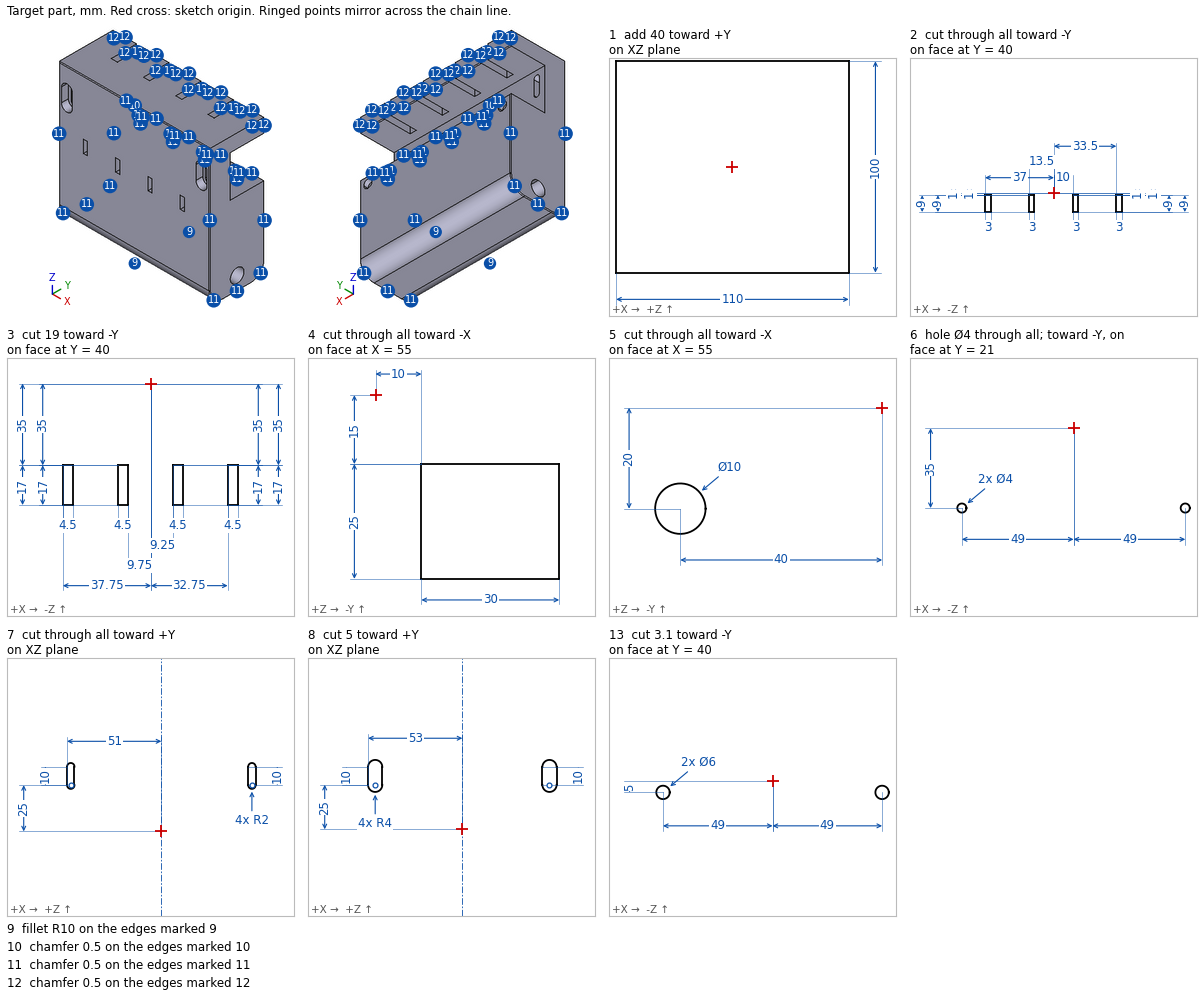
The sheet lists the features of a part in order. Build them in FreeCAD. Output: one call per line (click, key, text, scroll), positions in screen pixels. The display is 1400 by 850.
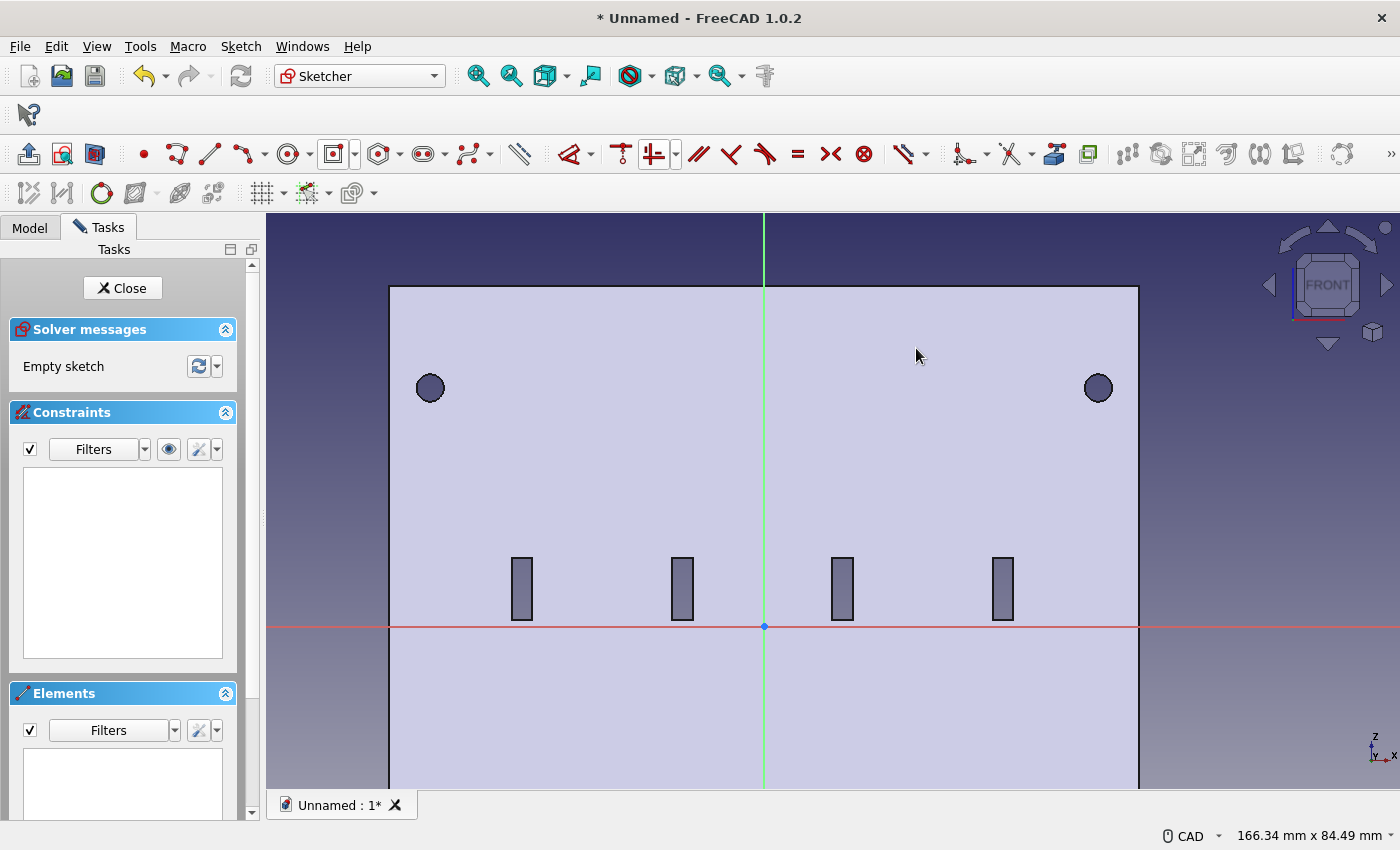
scroll(430, 456, up, 3)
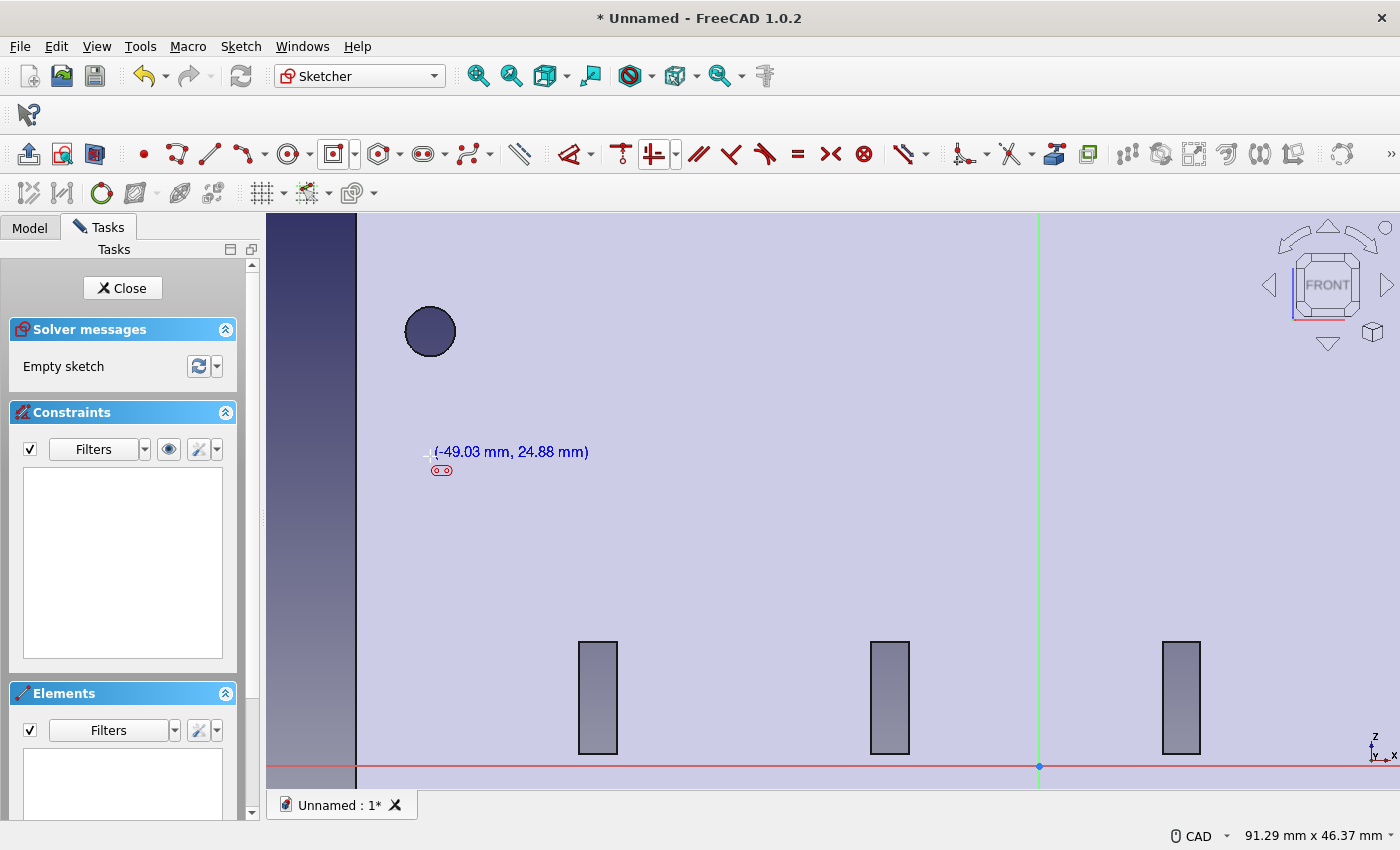
click(430, 456)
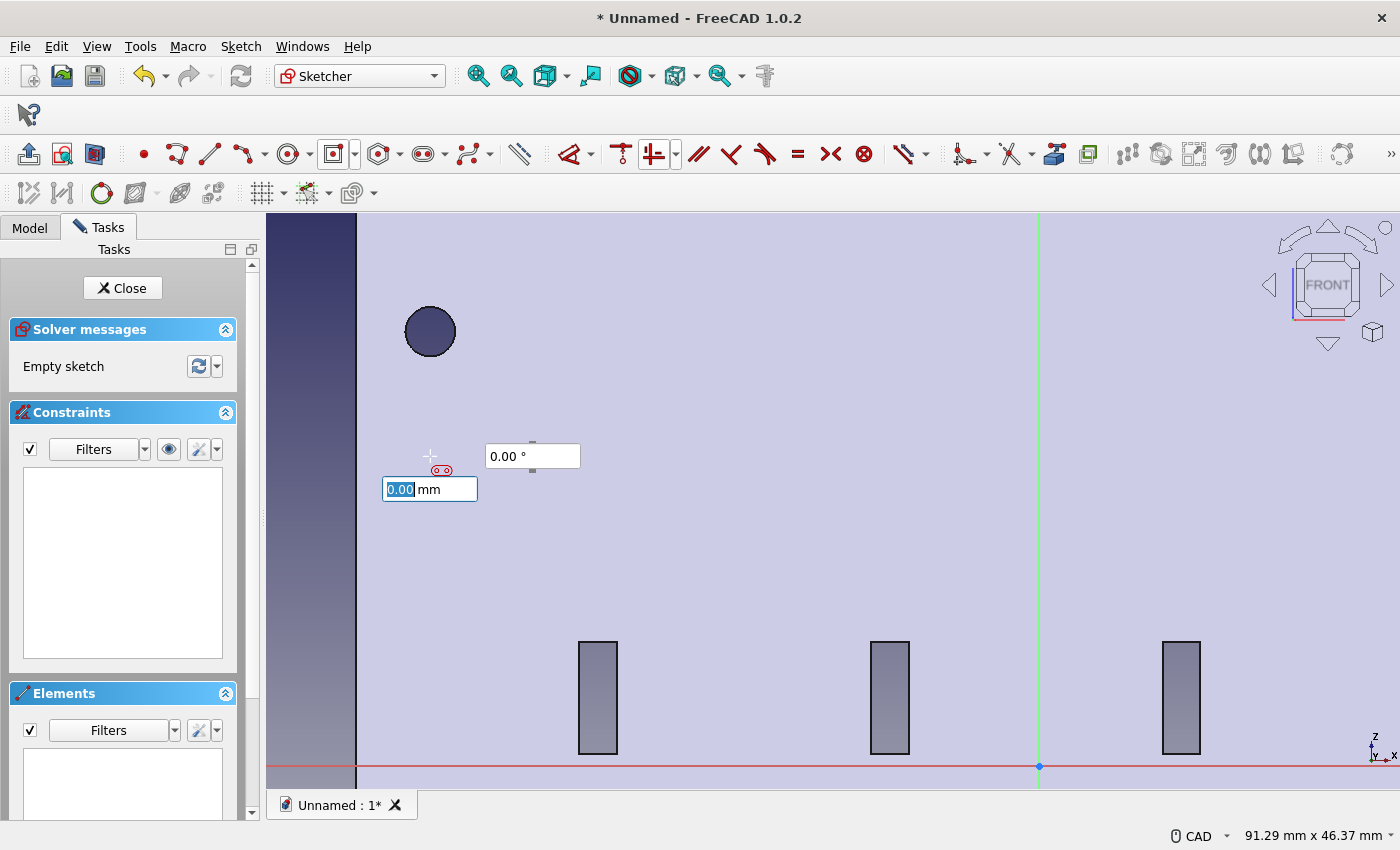
click(430, 332)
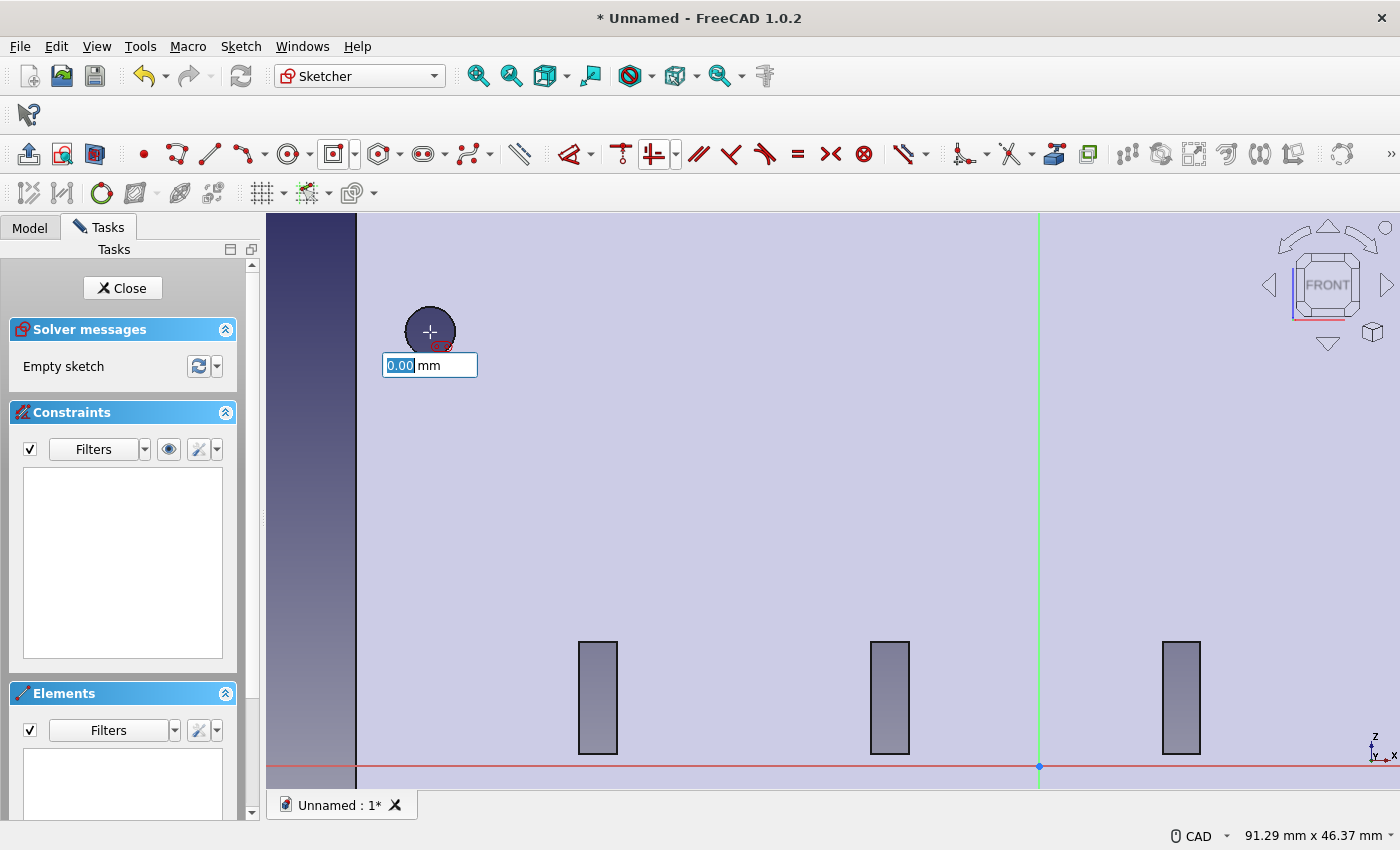
click(455, 394)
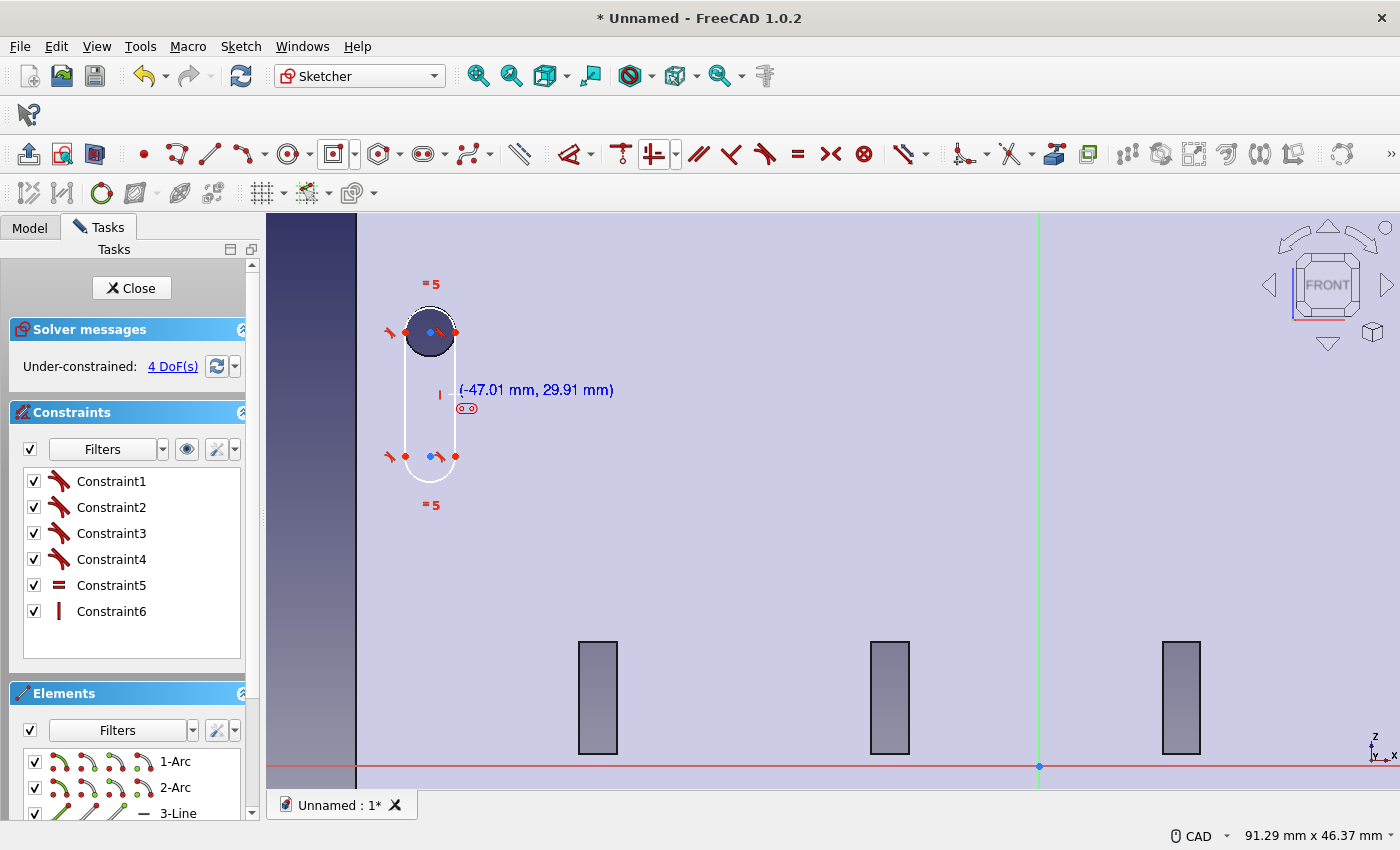
scroll(431, 458, down, 3)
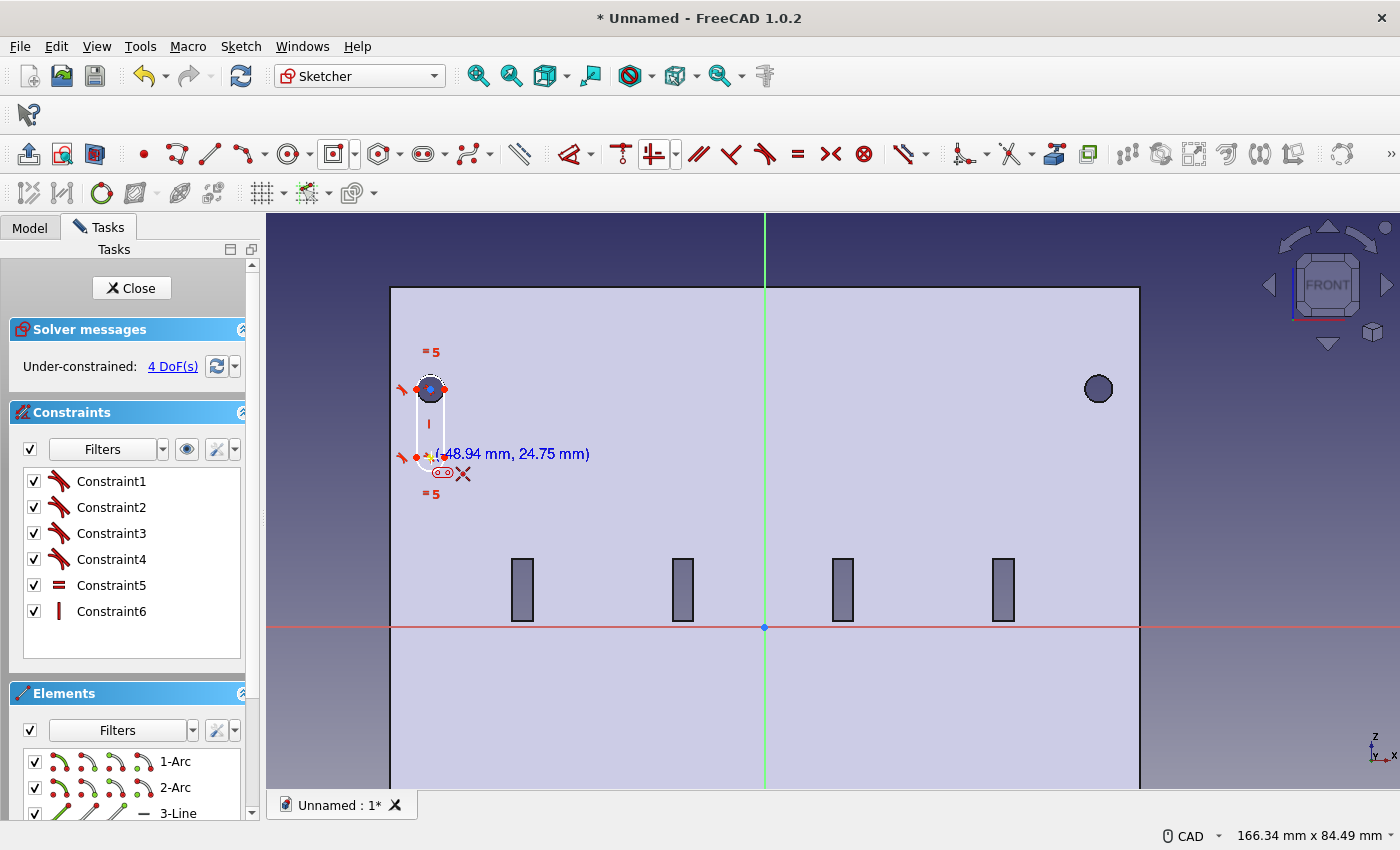
scroll(1099, 457, up, 3)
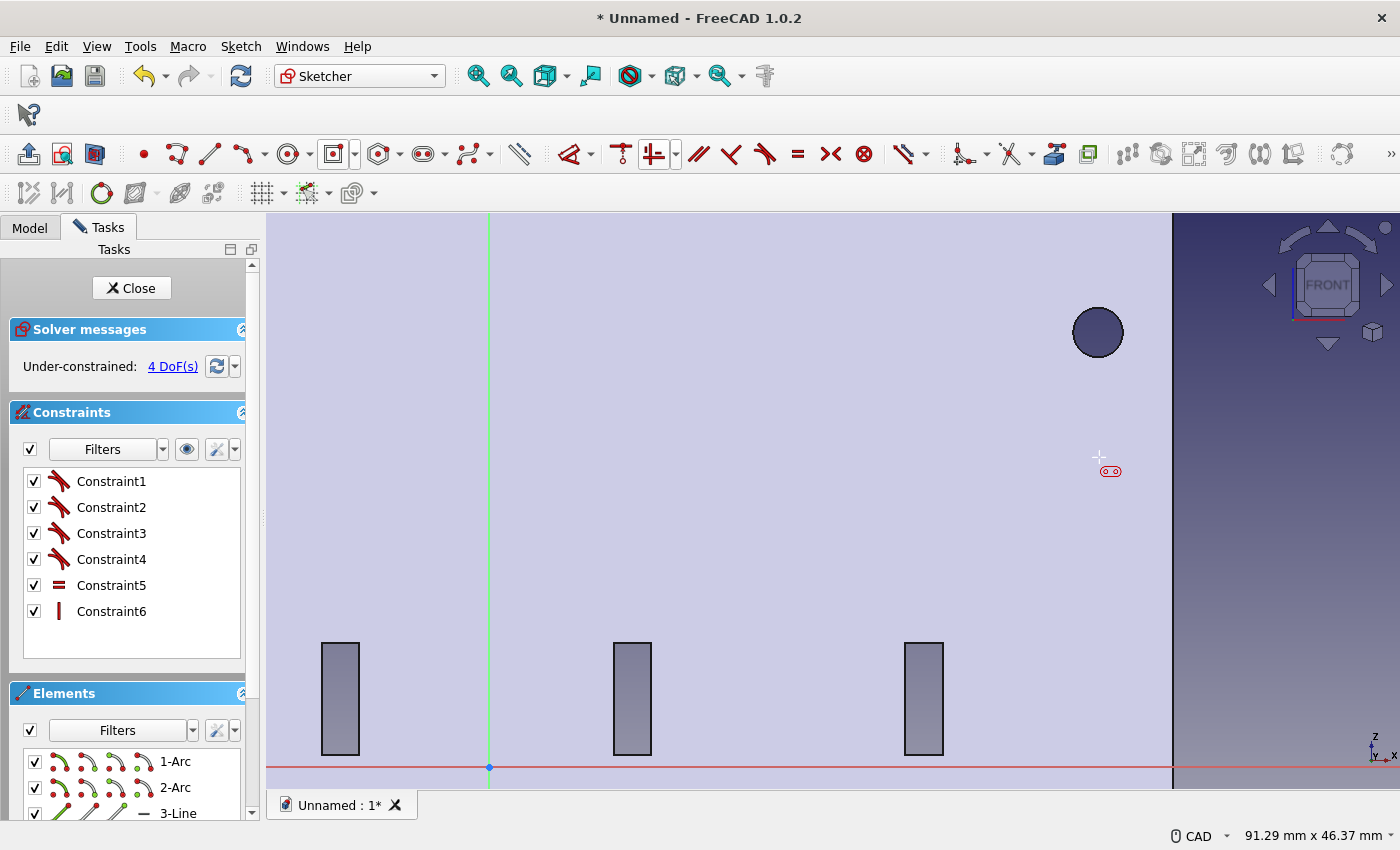
click(1098, 457)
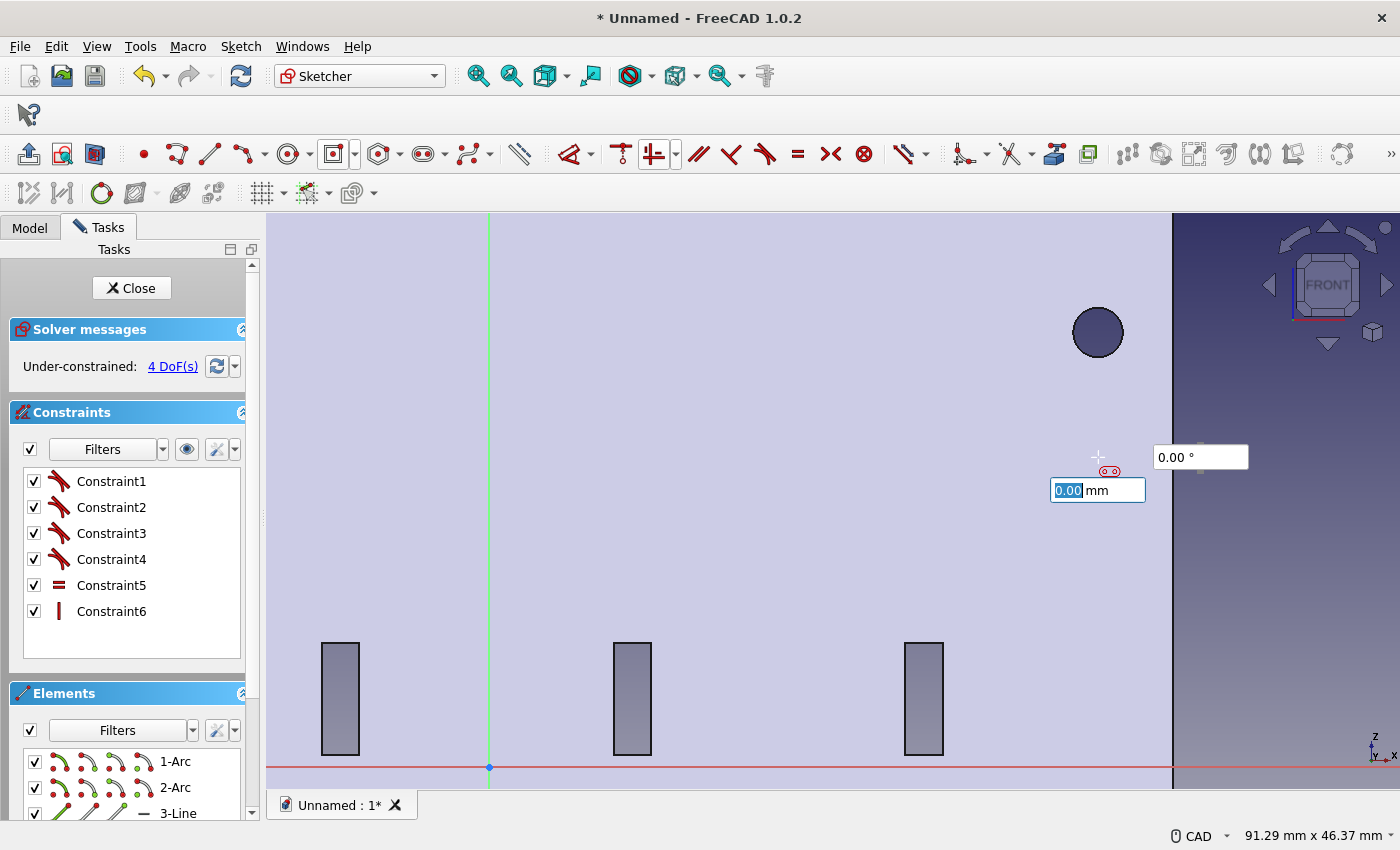
click(1098, 333)